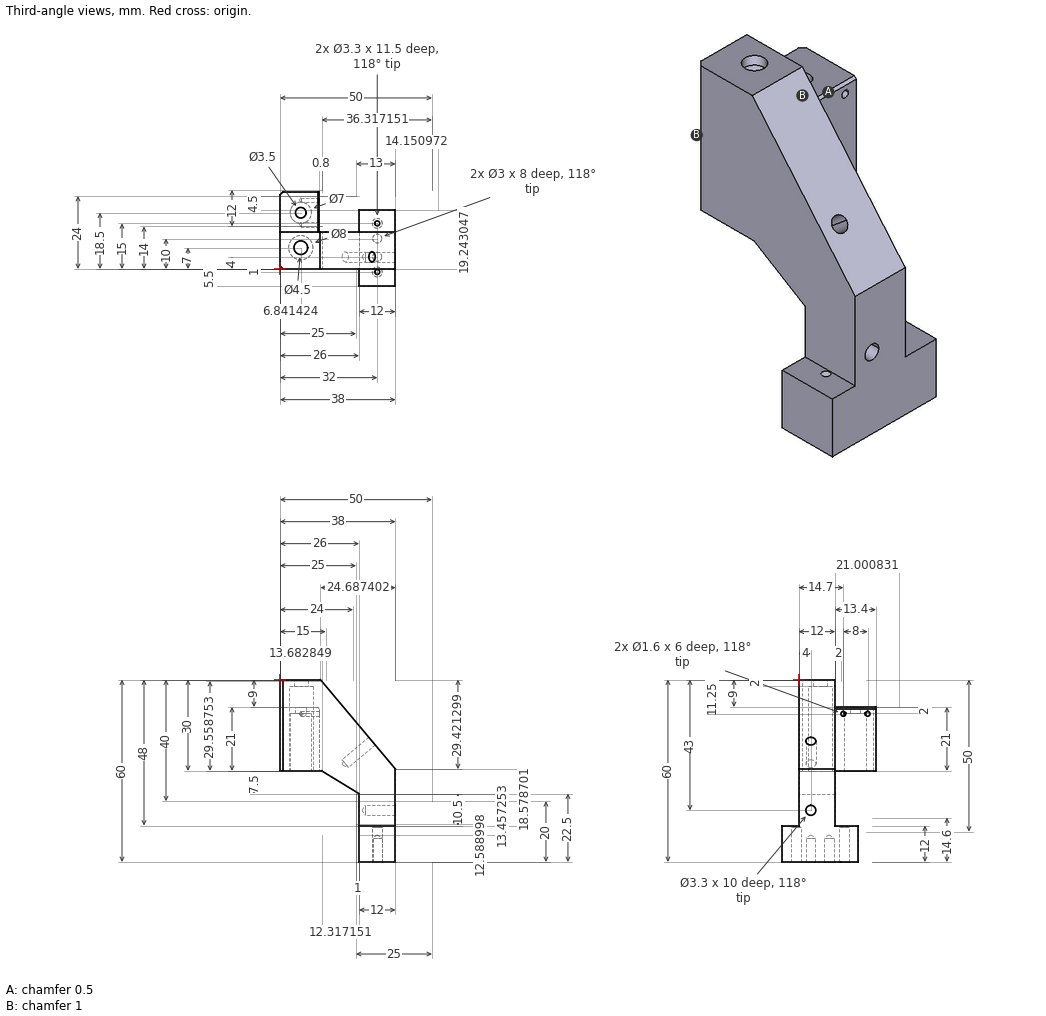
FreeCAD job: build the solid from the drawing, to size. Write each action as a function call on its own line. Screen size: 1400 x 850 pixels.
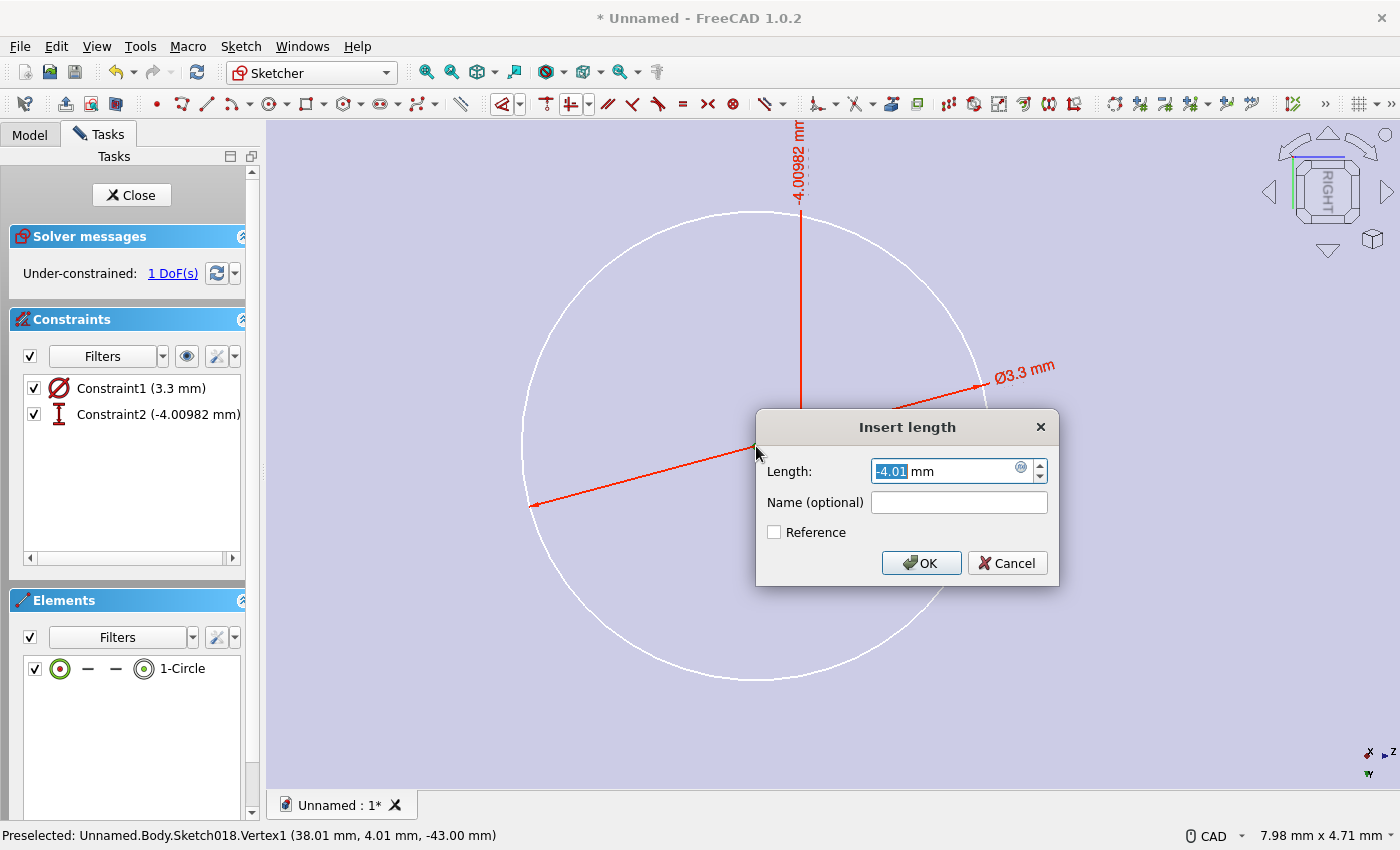
text(-4)
key(Return)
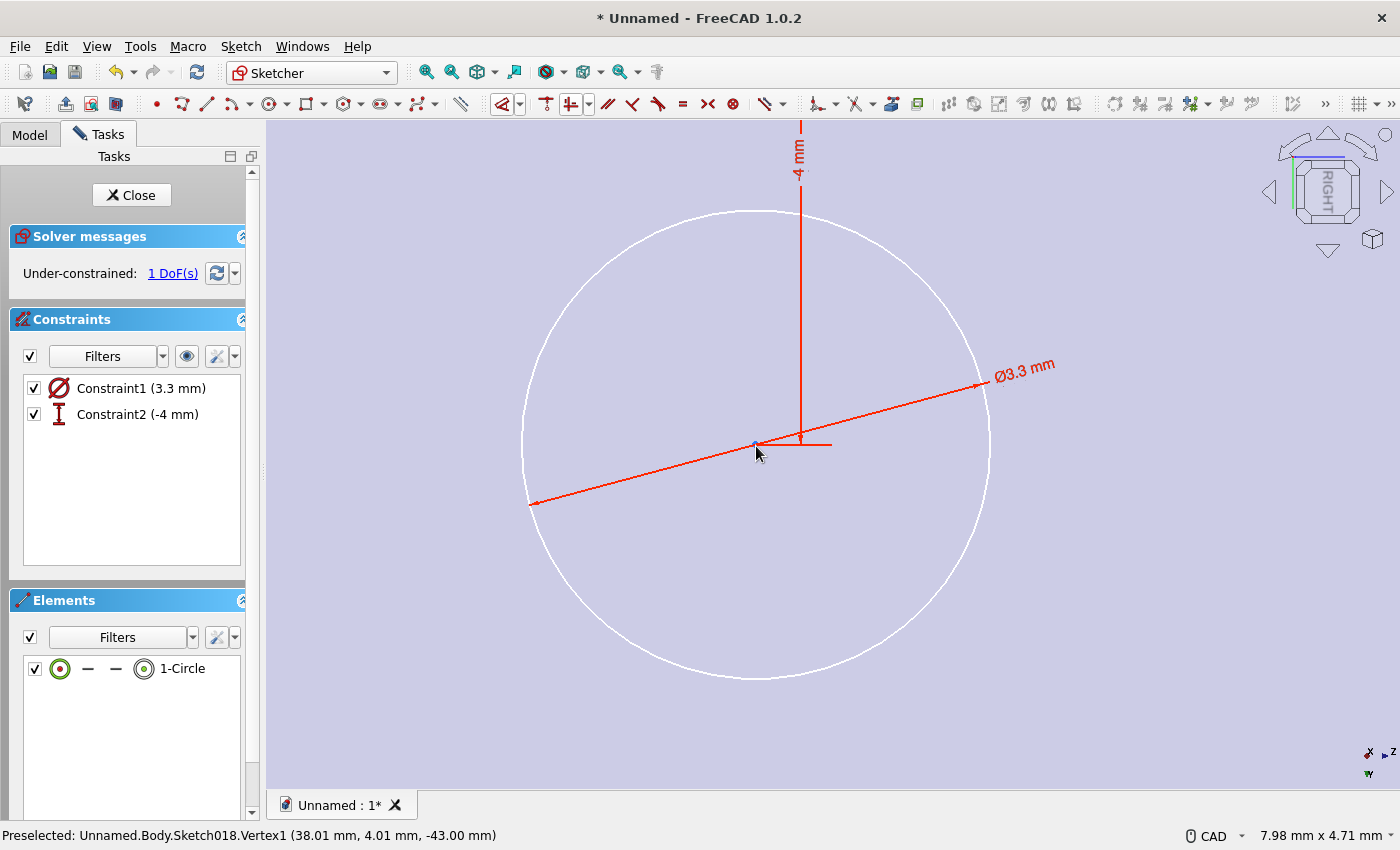
click(756, 445)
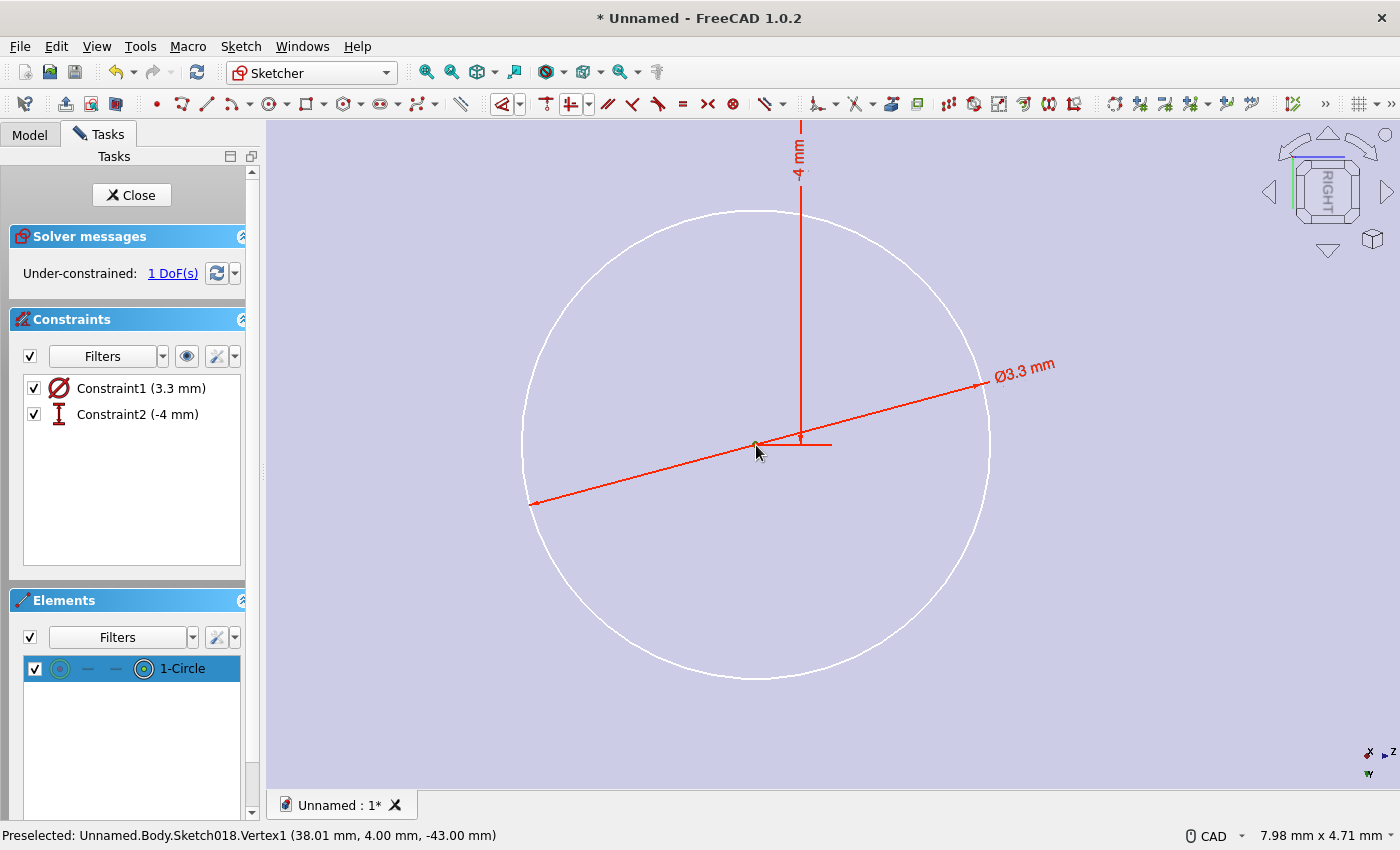
key(l)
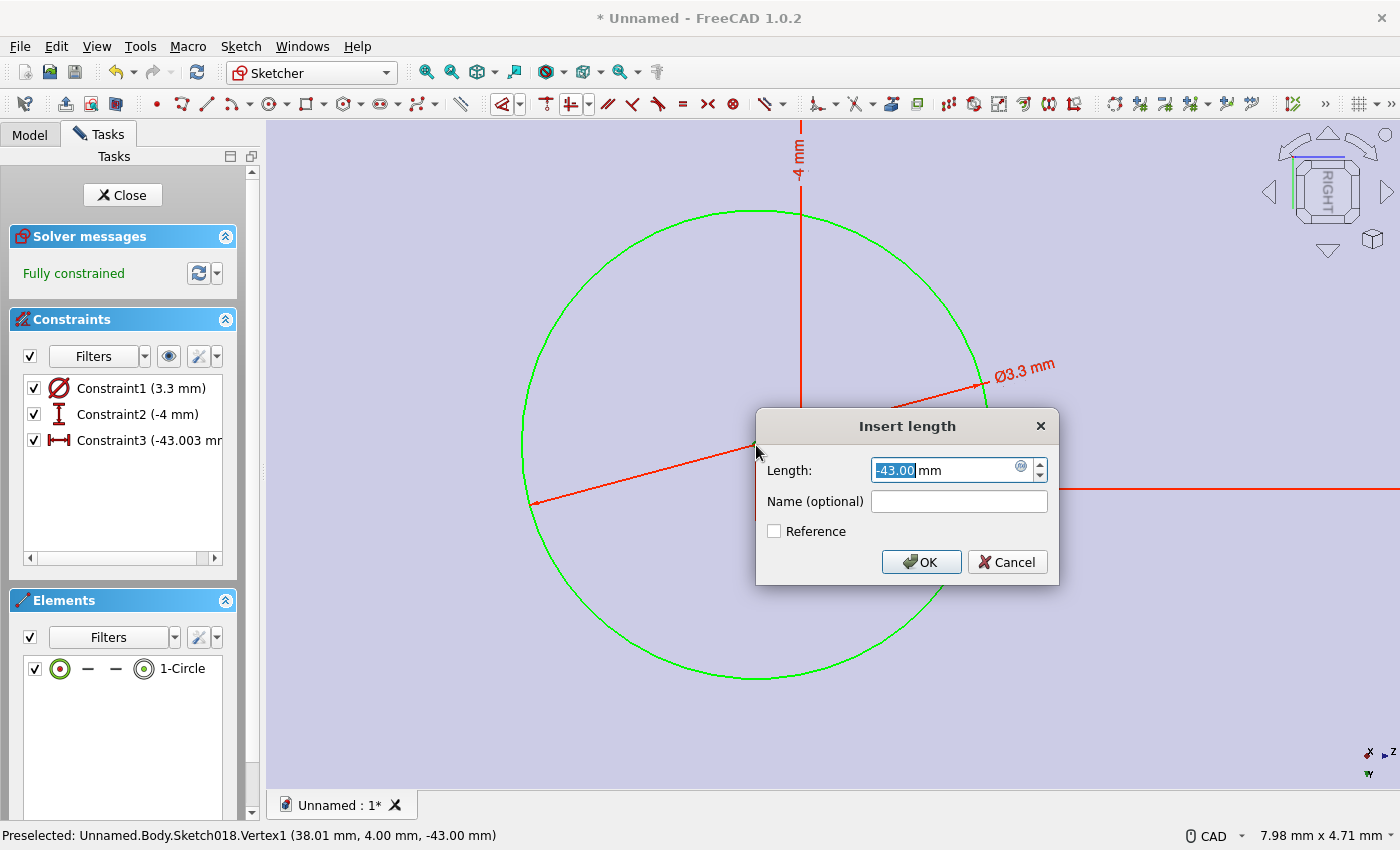
text(-43)
key(Return)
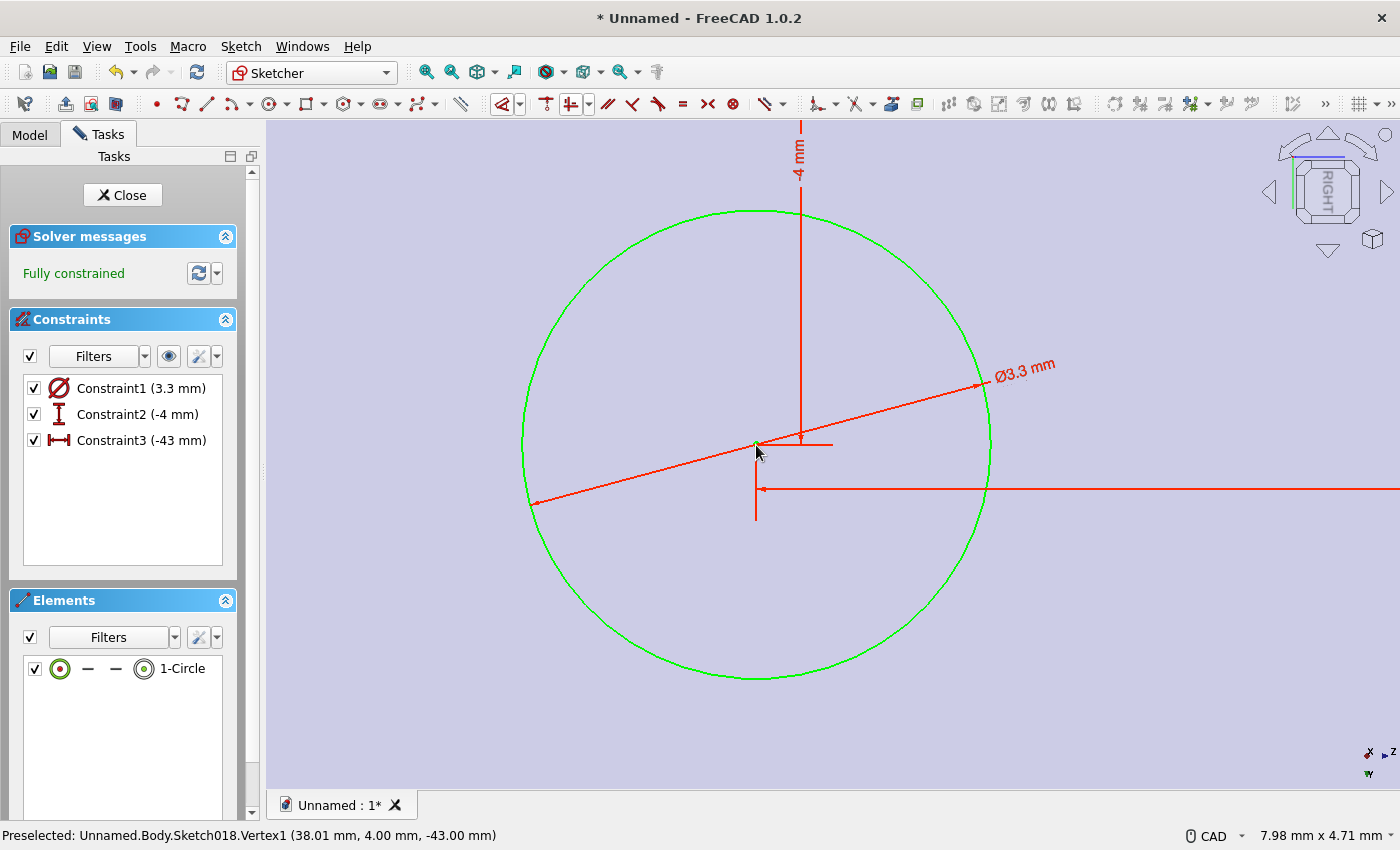
click(123, 195)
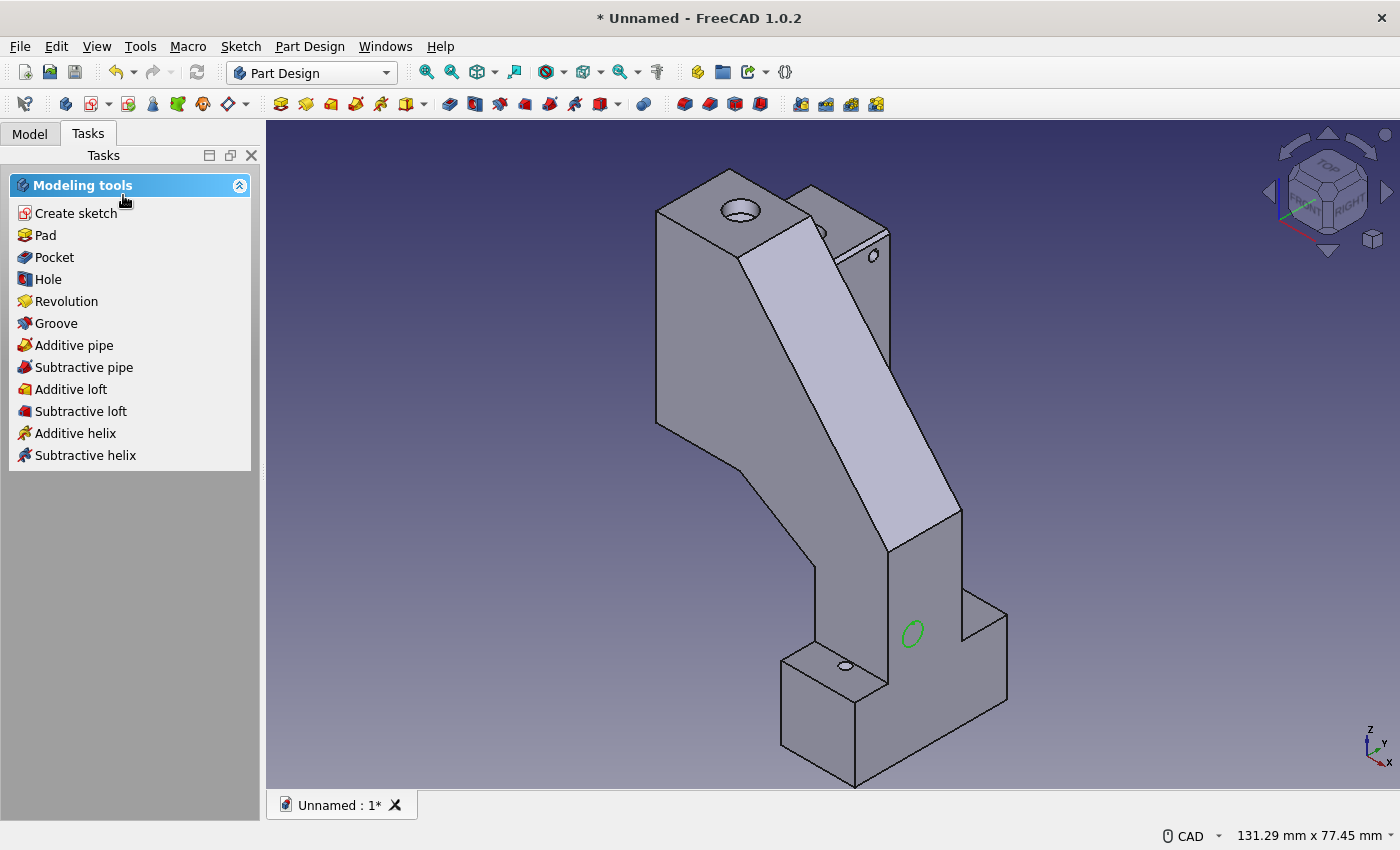
click(475, 104)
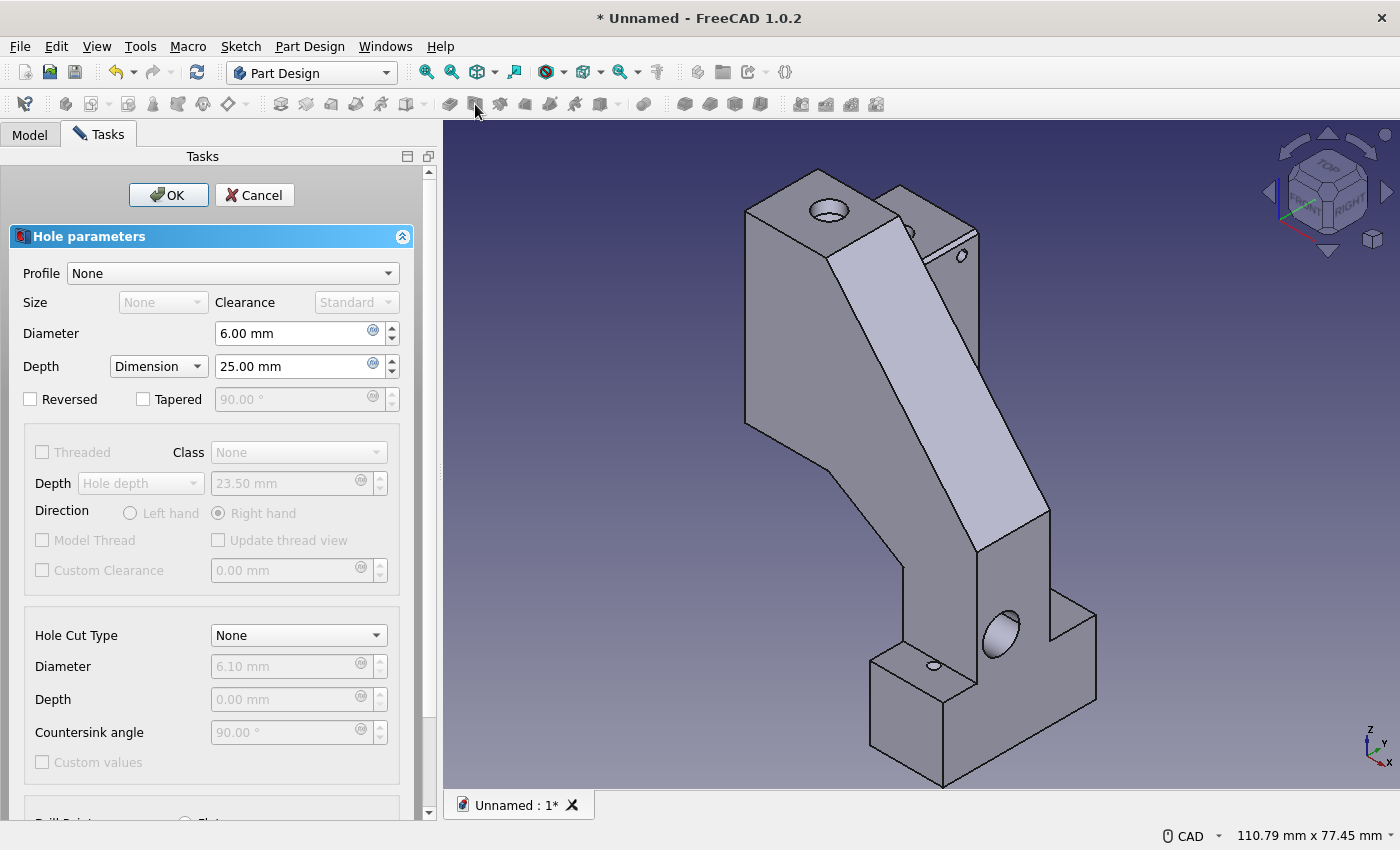
triple_click(300, 334)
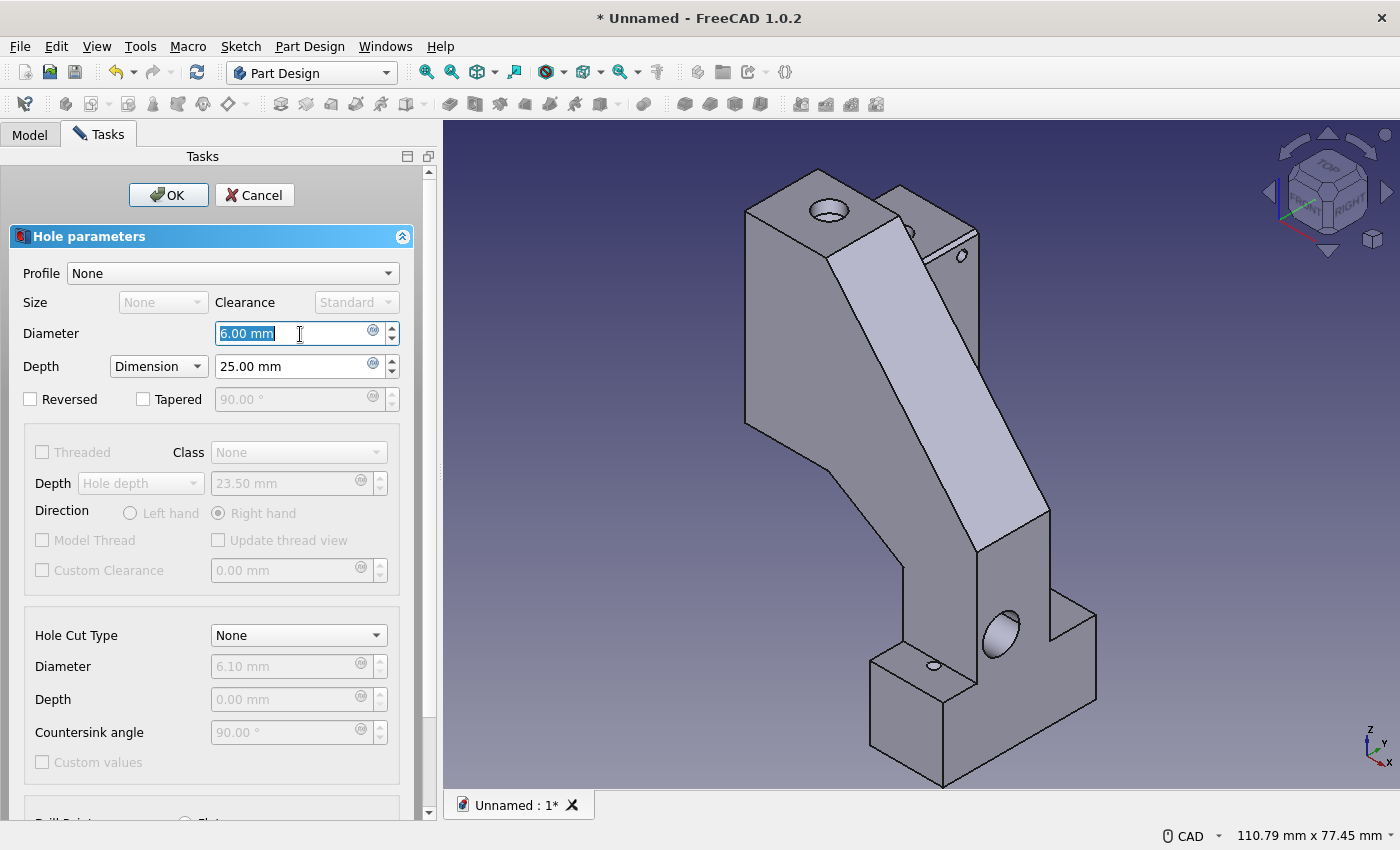
text(3.3)
key(Tab)